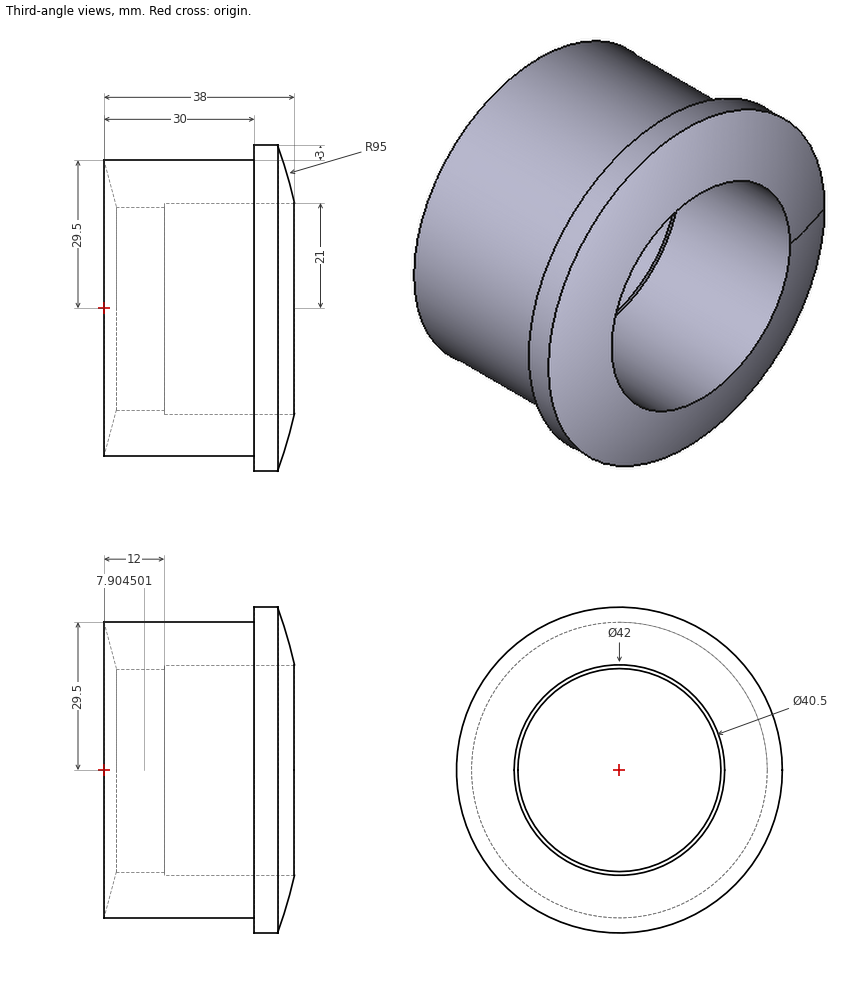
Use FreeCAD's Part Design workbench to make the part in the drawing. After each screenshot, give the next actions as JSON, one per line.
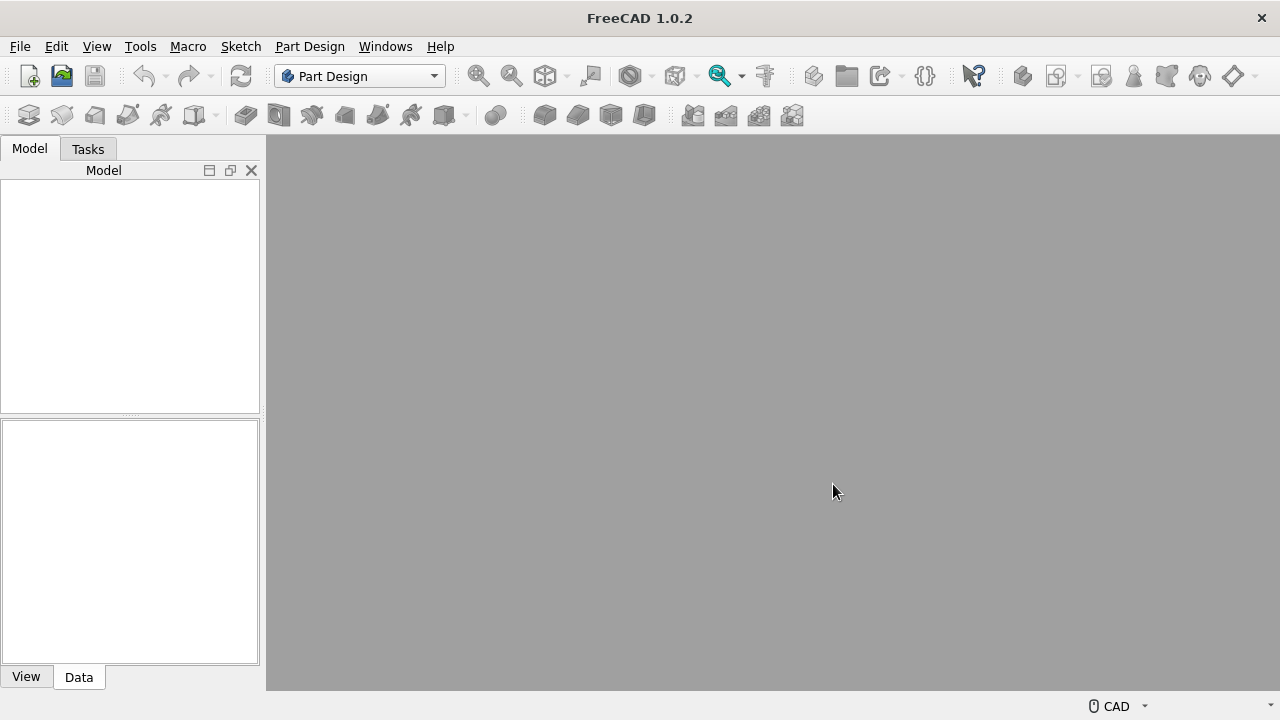
{"action": "left_click", "coordinate": [29, 76]}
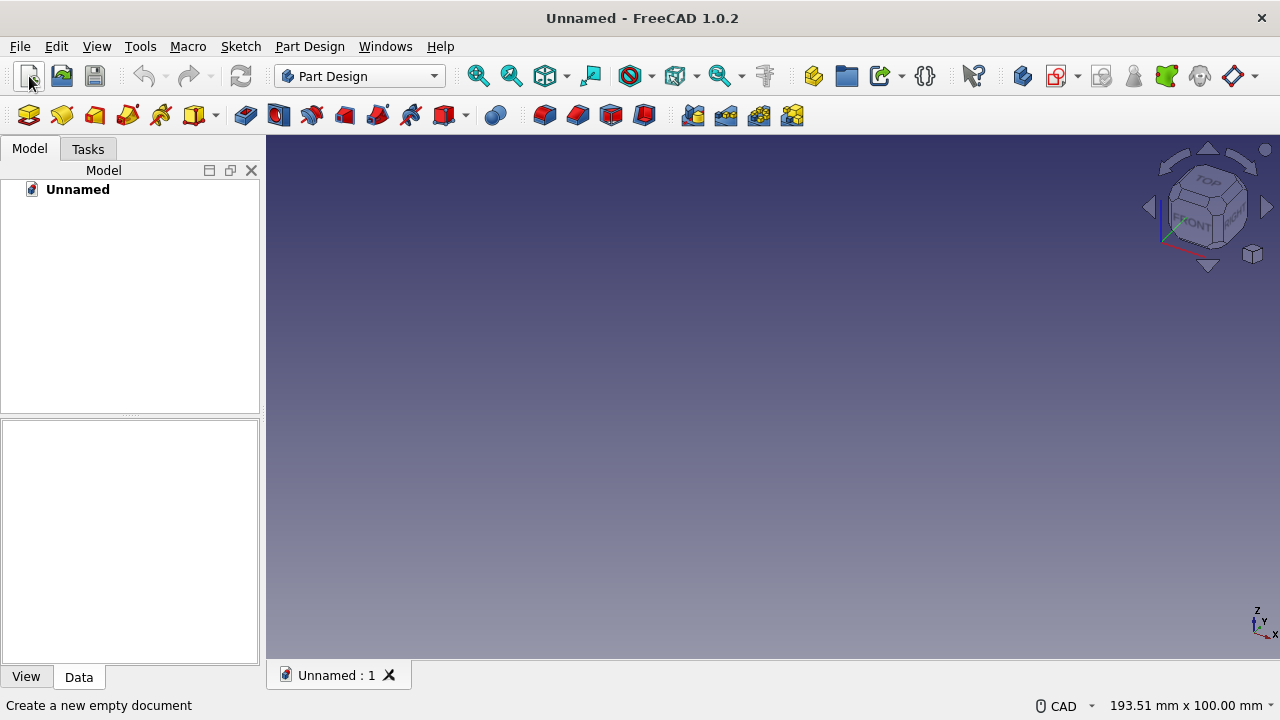
{"action": "left_click", "coordinate": [1056, 76]}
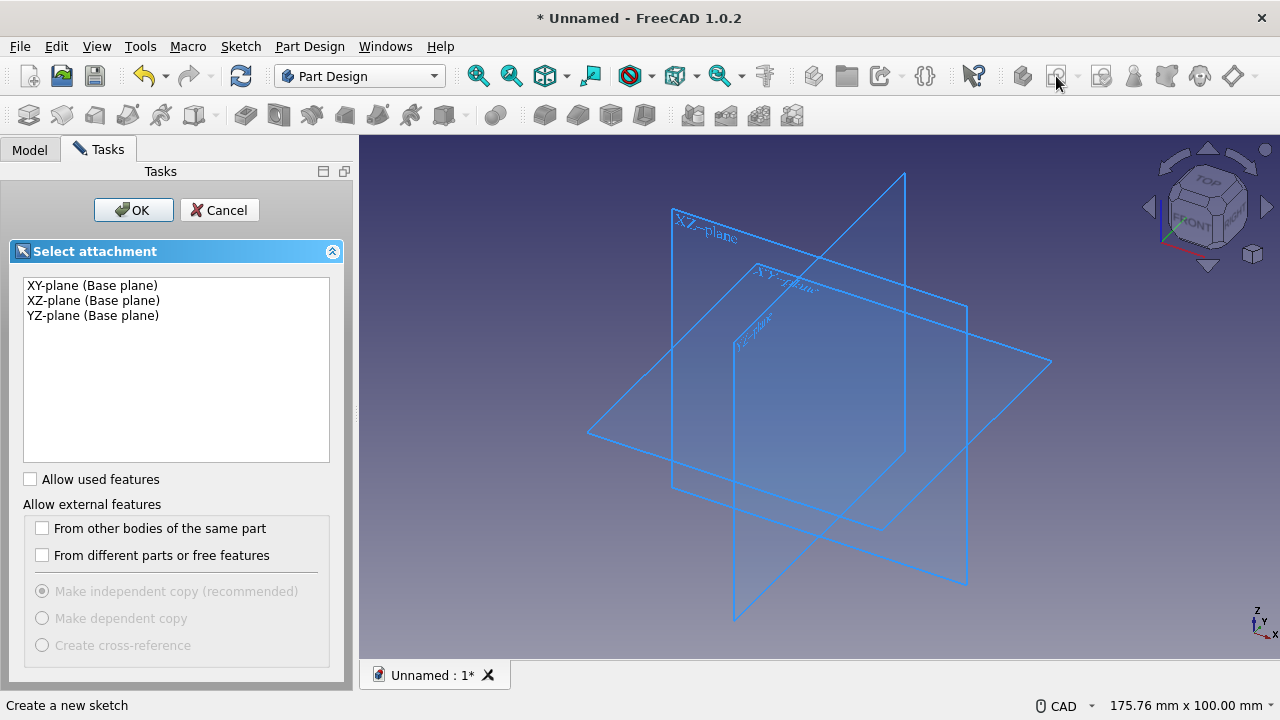
{"action": "left_click", "coordinate": [84, 286]}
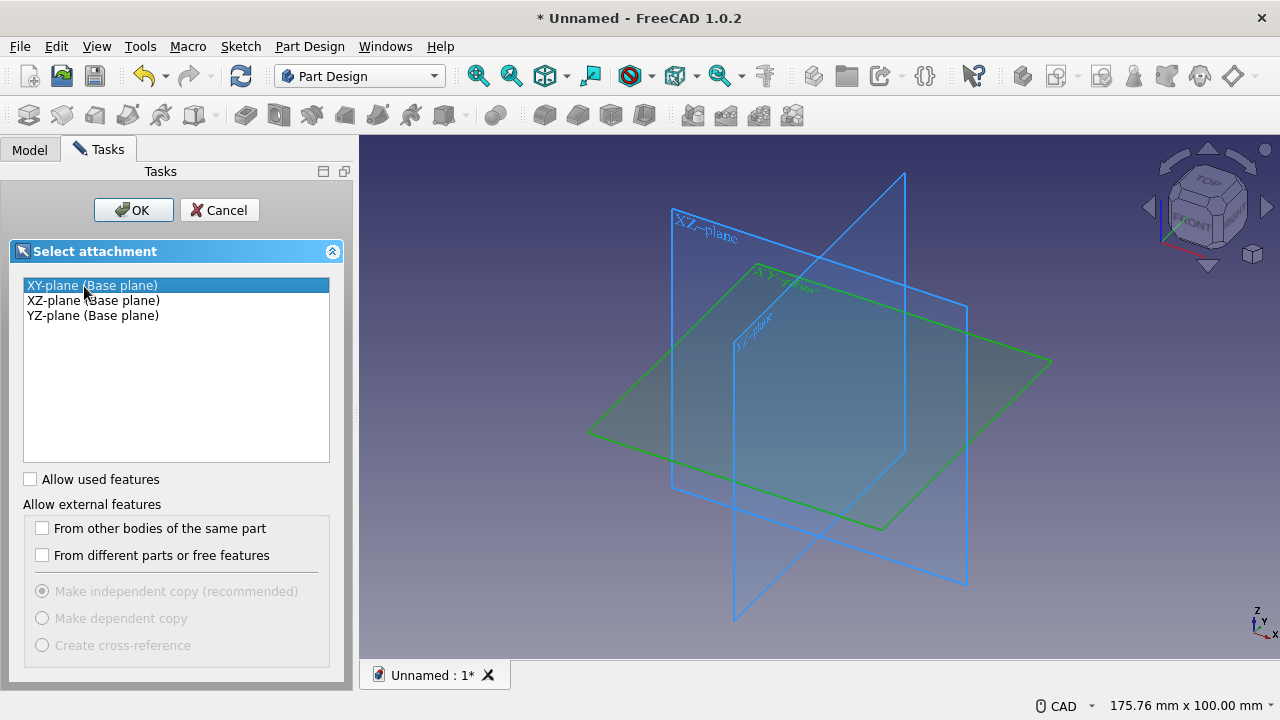
{"action": "left_click", "coordinate": [134, 210]}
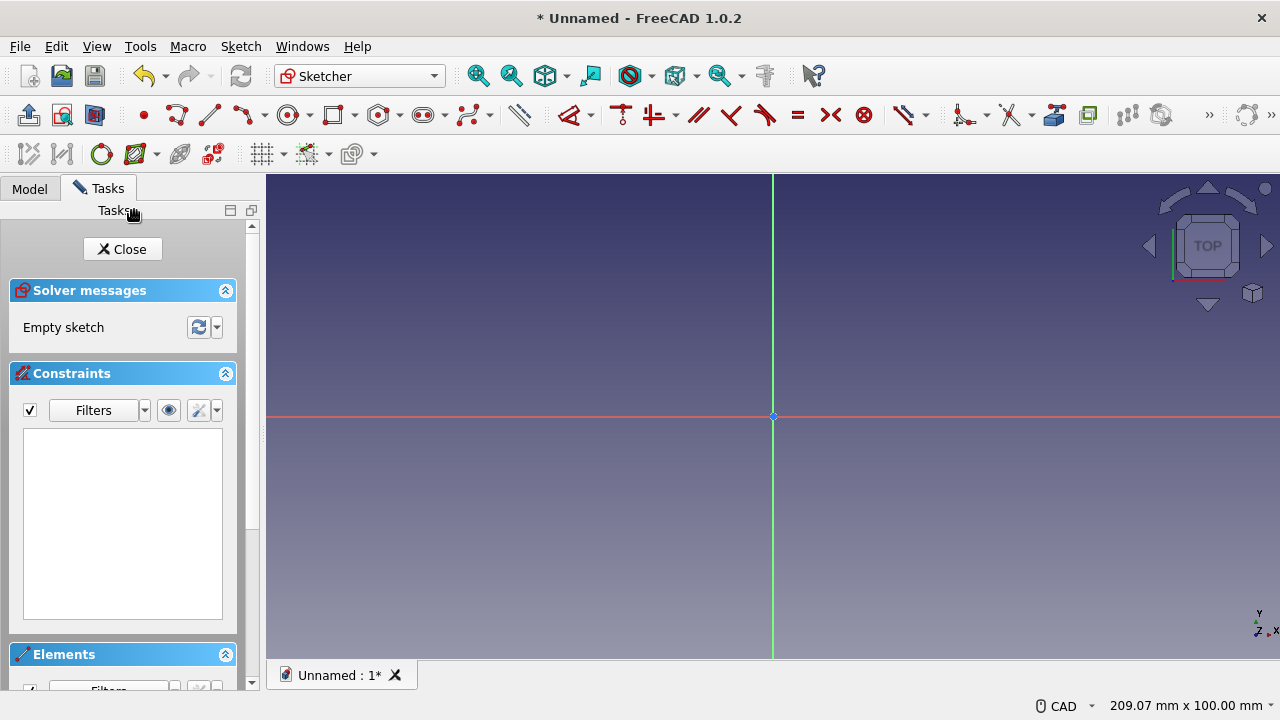
{"action": "scroll", "coordinate": [1061, 242], "scroll_direction": "up", "scroll_amount": 3}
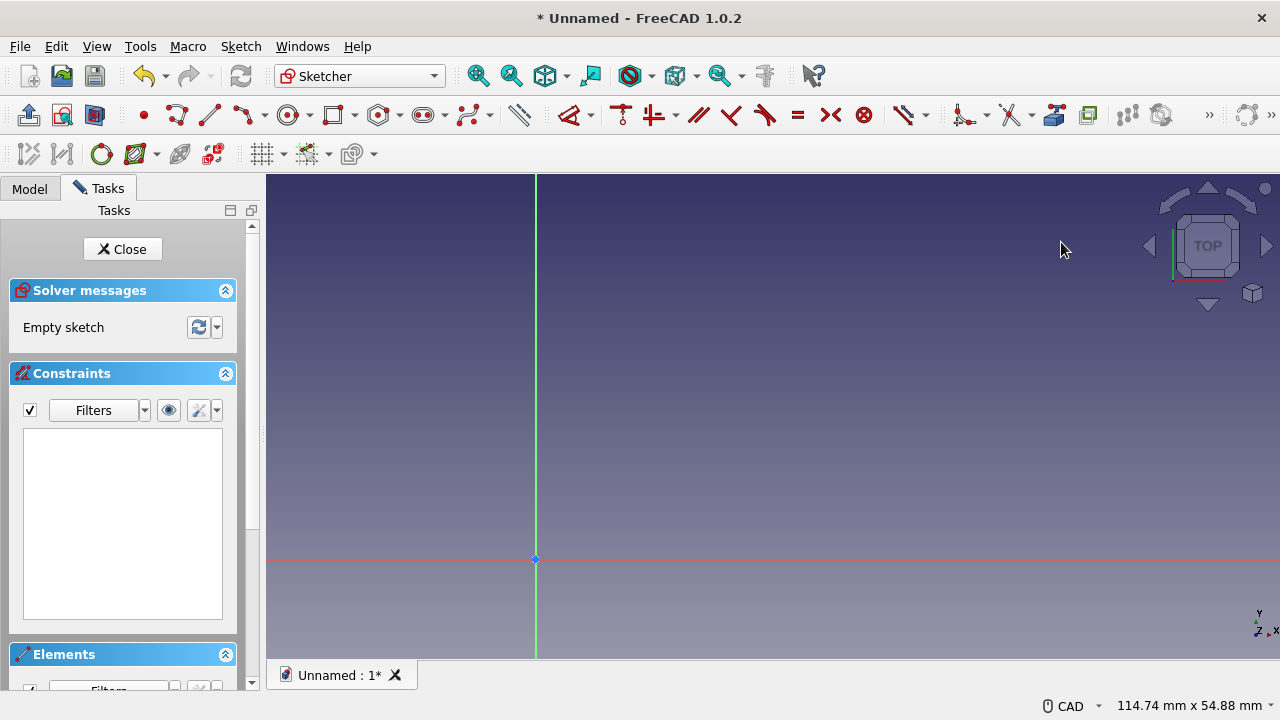
{"action": "left_click", "coordinate": [177, 116]}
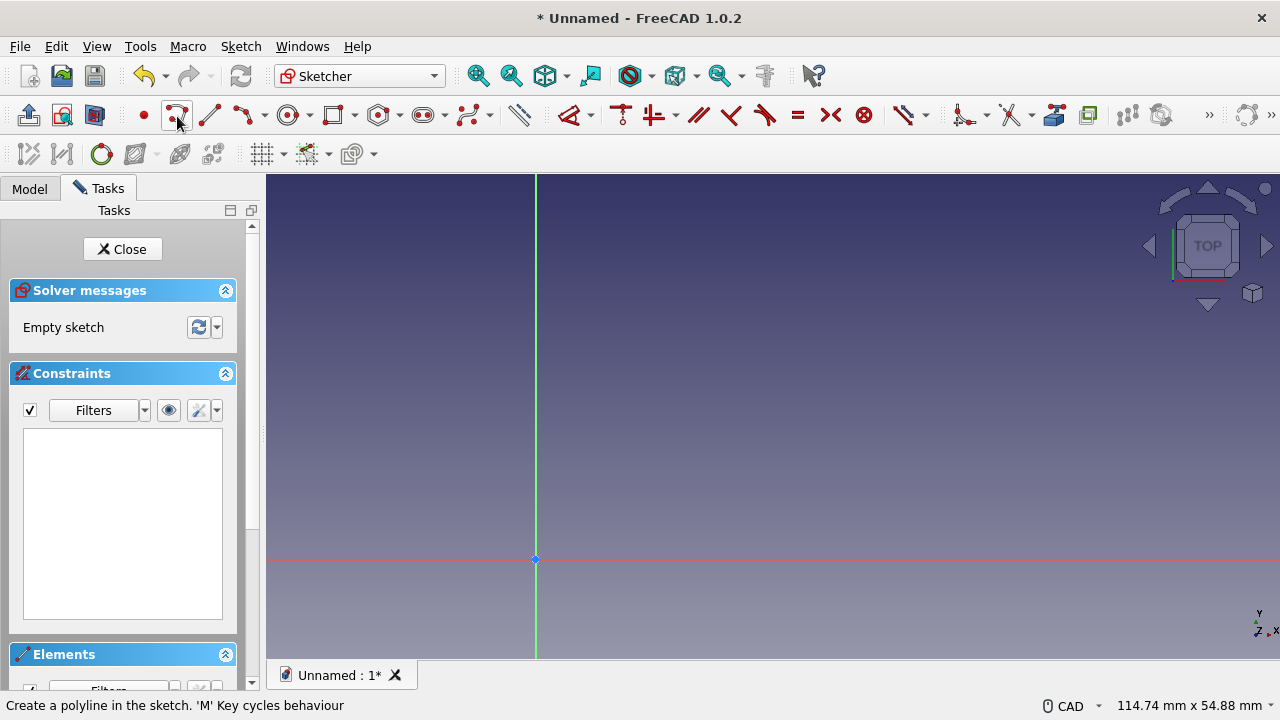
{"action": "left_click", "coordinate": [842, 273]}
{"action": "left_click", "coordinate": [801, 273]}
{"action": "left_click", "coordinate": [801, 299]}
{"action": "left_click", "coordinate": [536, 299]}
{"action": "left_click", "coordinate": [536, 560]}
{"action": "left_click", "coordinate": [871, 551]}
{"action": "left_click", "coordinate": [871, 374]}
{"action": "right_click", "coordinate": [871, 374]}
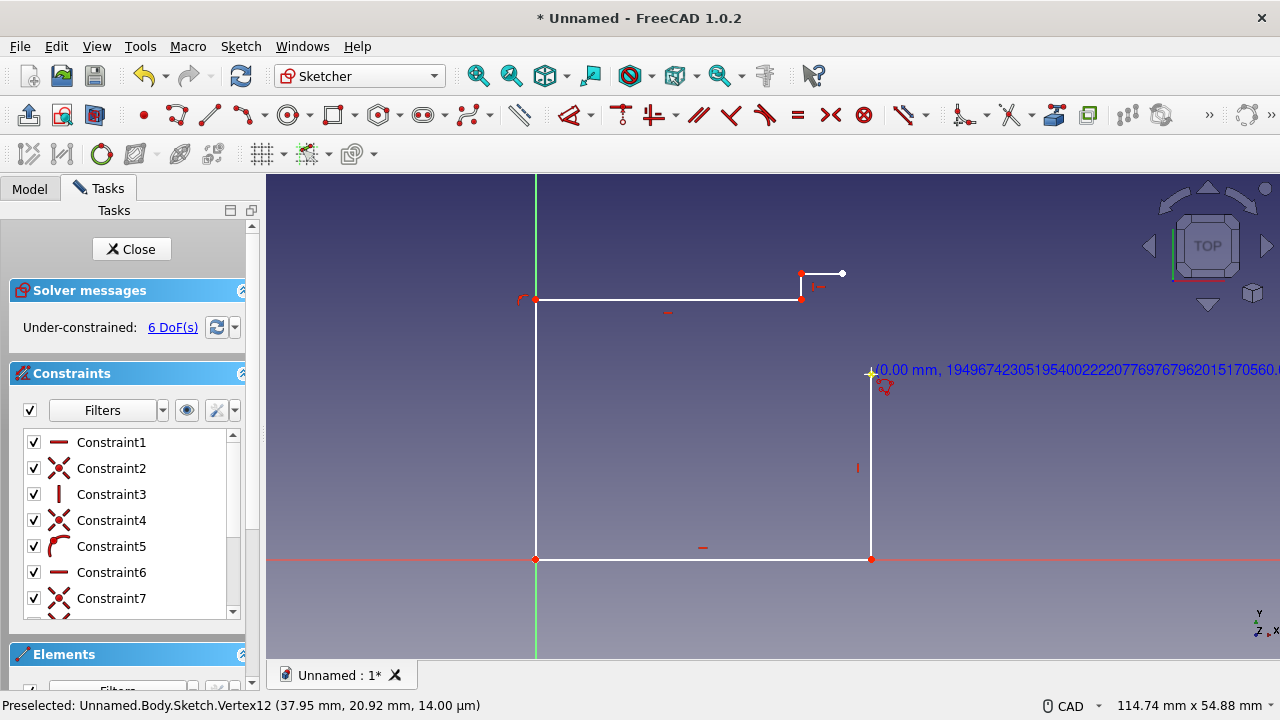
{"action": "left_click", "coordinate": [242, 116]}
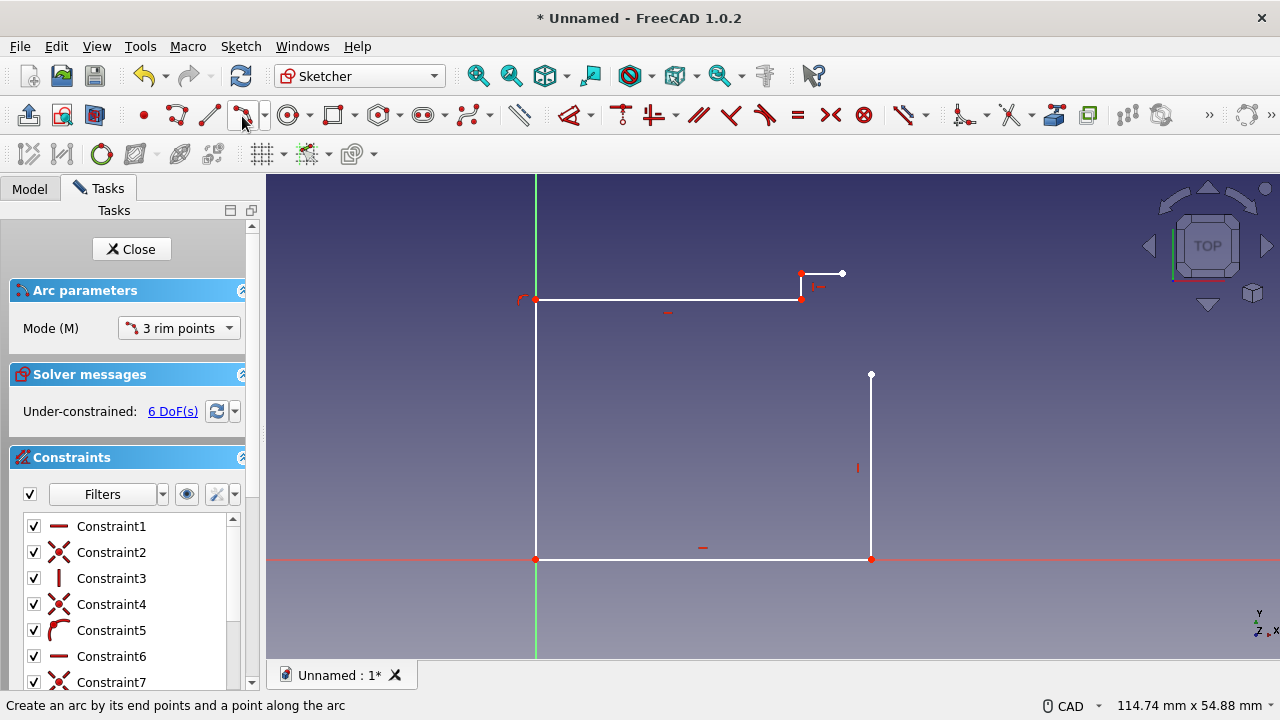
{"action": "left_click", "coordinate": [871, 375]}
{"action": "left_click", "coordinate": [842, 274]}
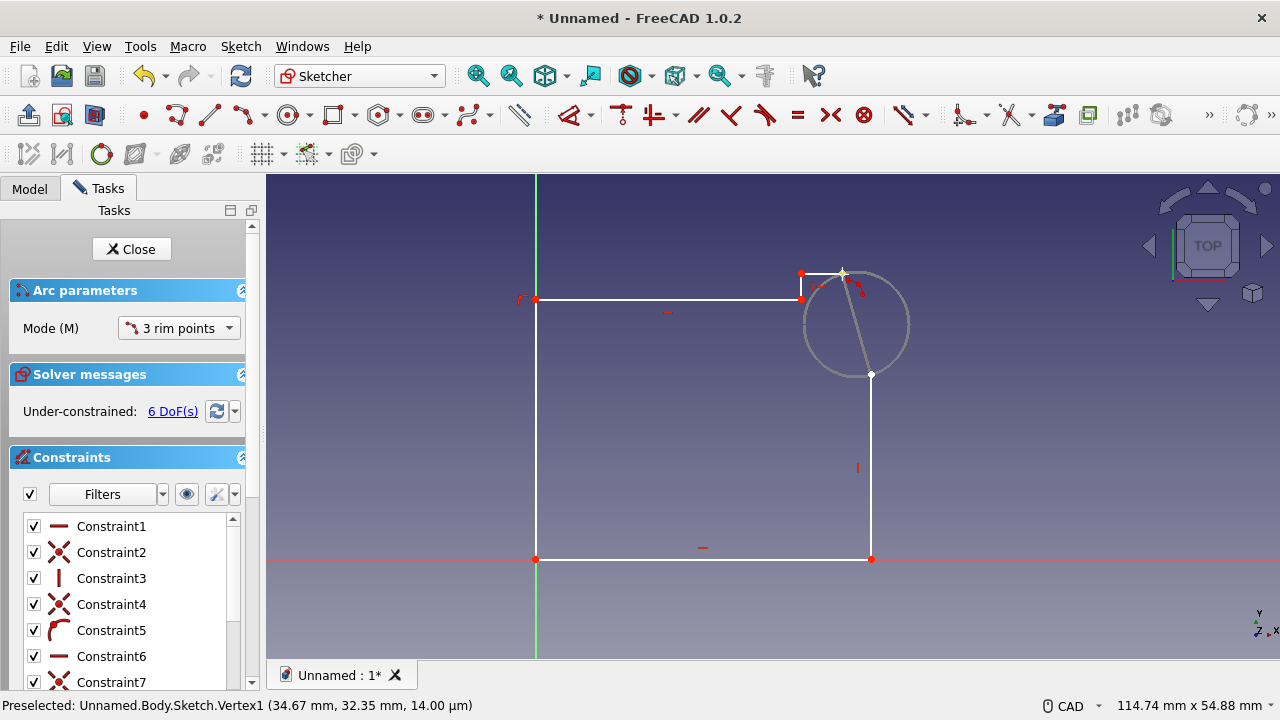
{"action": "scroll", "coordinate": [858, 323], "scroll_direction": "up", "scroll_amount": 12}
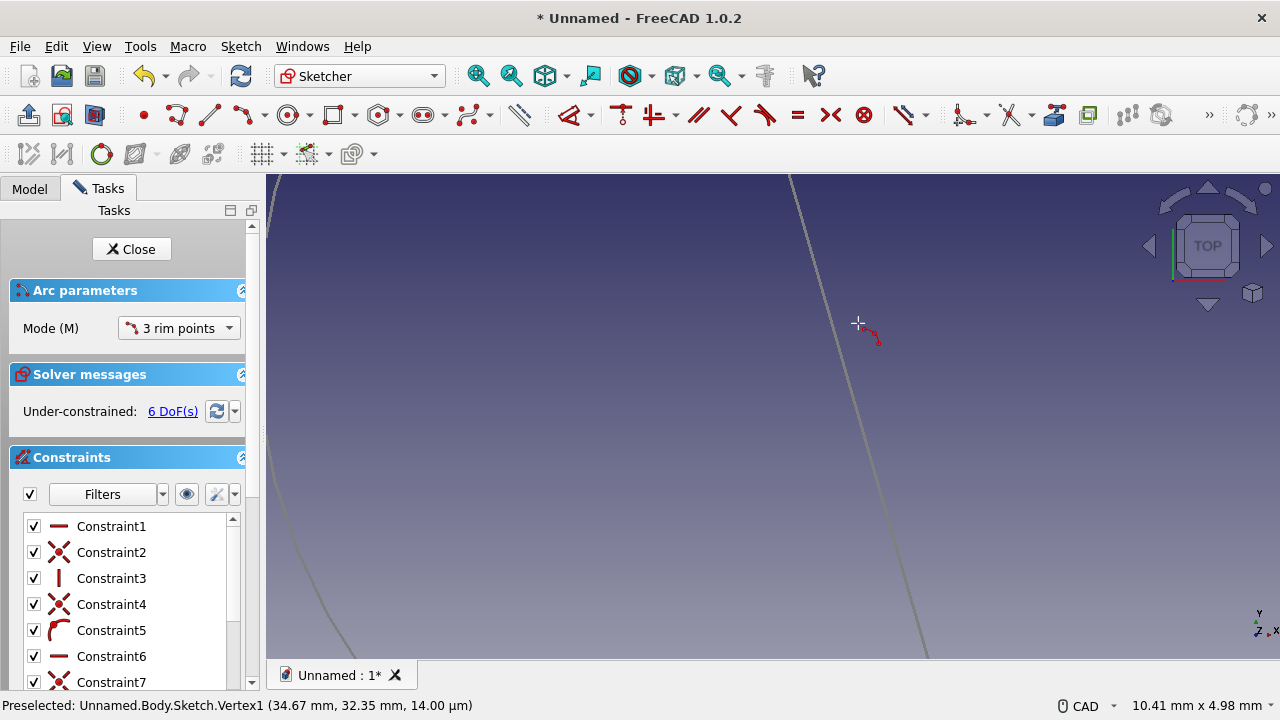
{"action": "left_click", "coordinate": [853, 320]}
{"action": "key", "text": "Escape"}